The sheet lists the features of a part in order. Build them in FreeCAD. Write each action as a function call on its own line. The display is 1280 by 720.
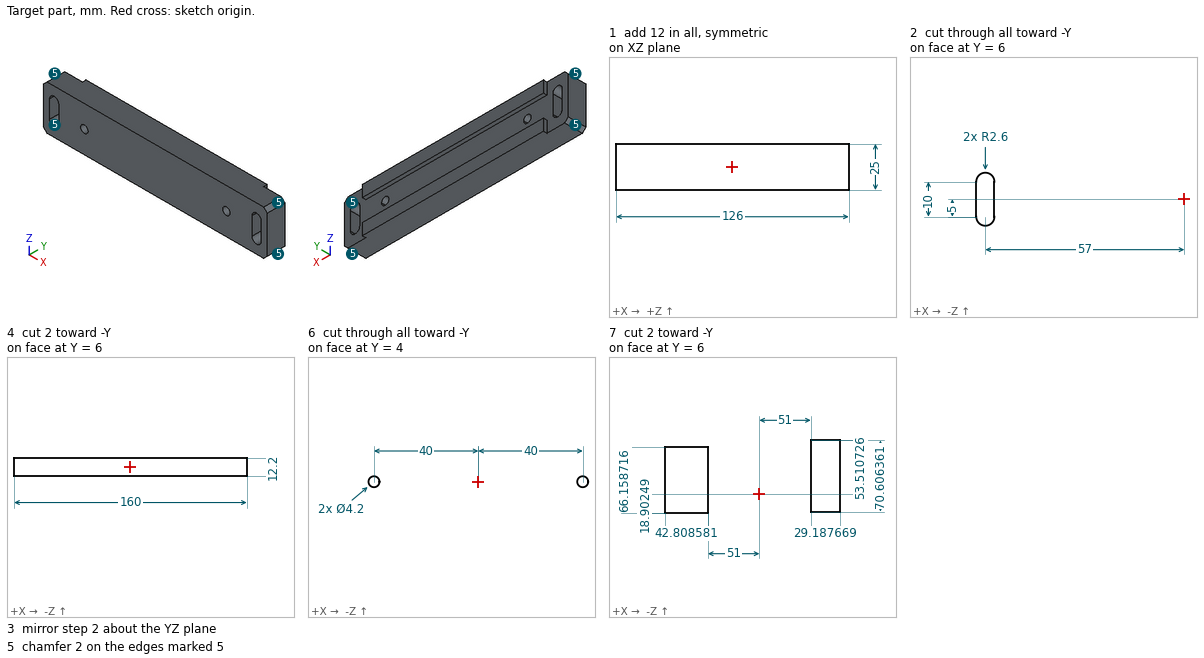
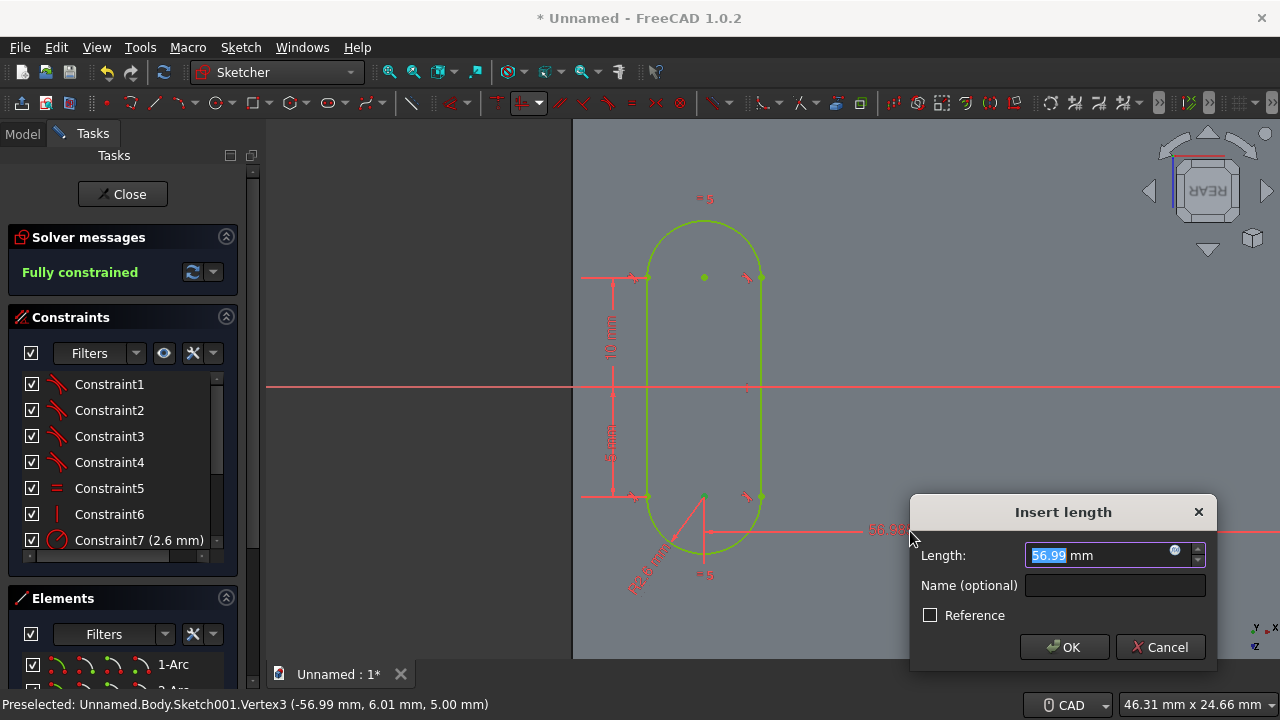
text(57)
key(Return)
key(Escape)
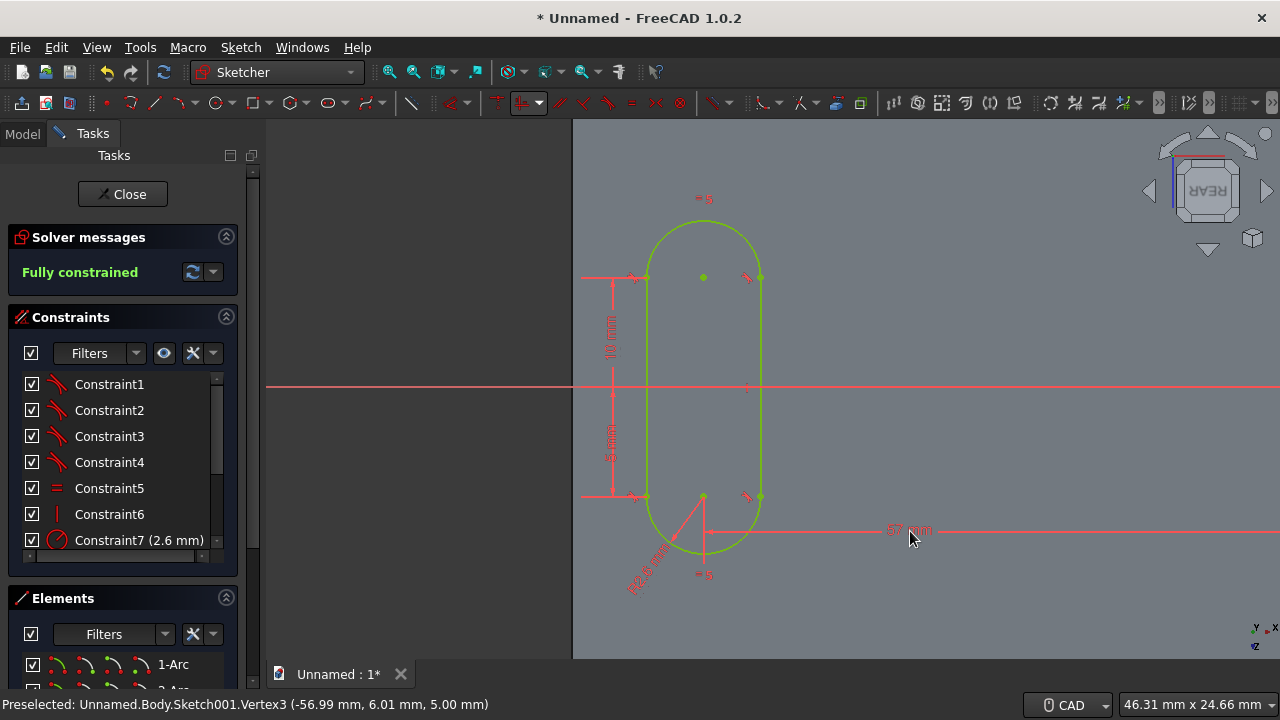
click(123, 194)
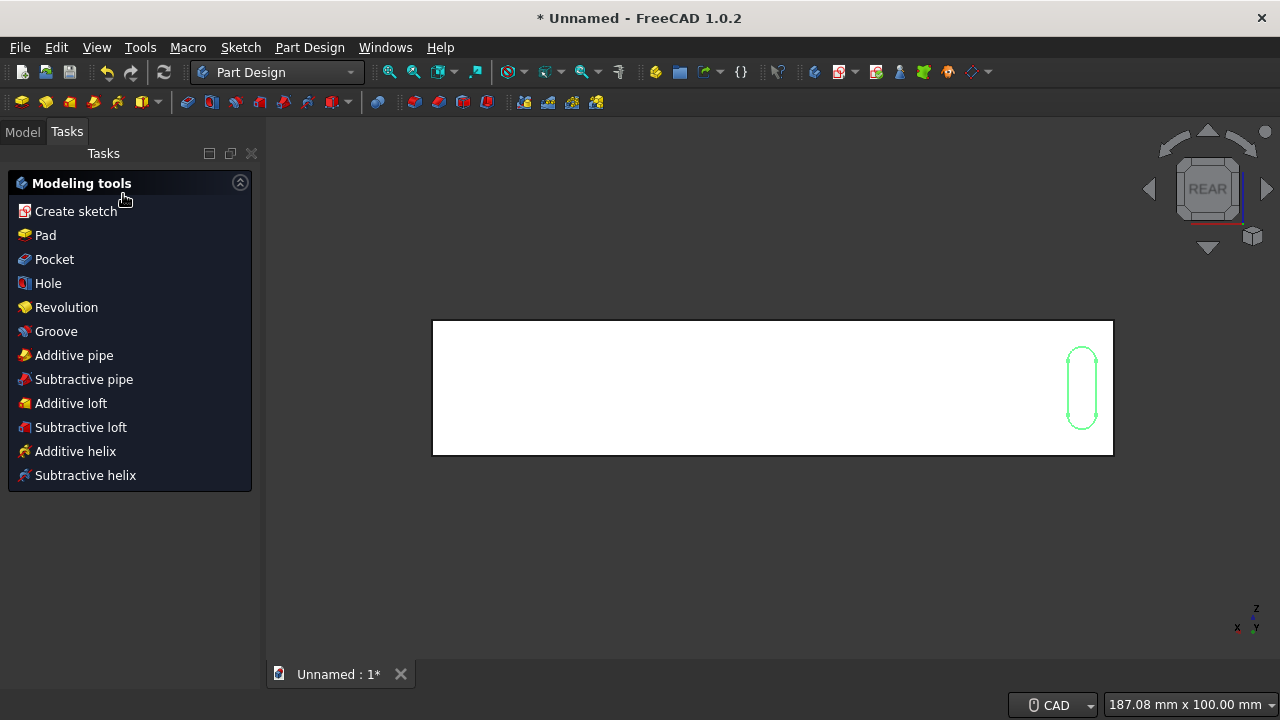
click(188, 102)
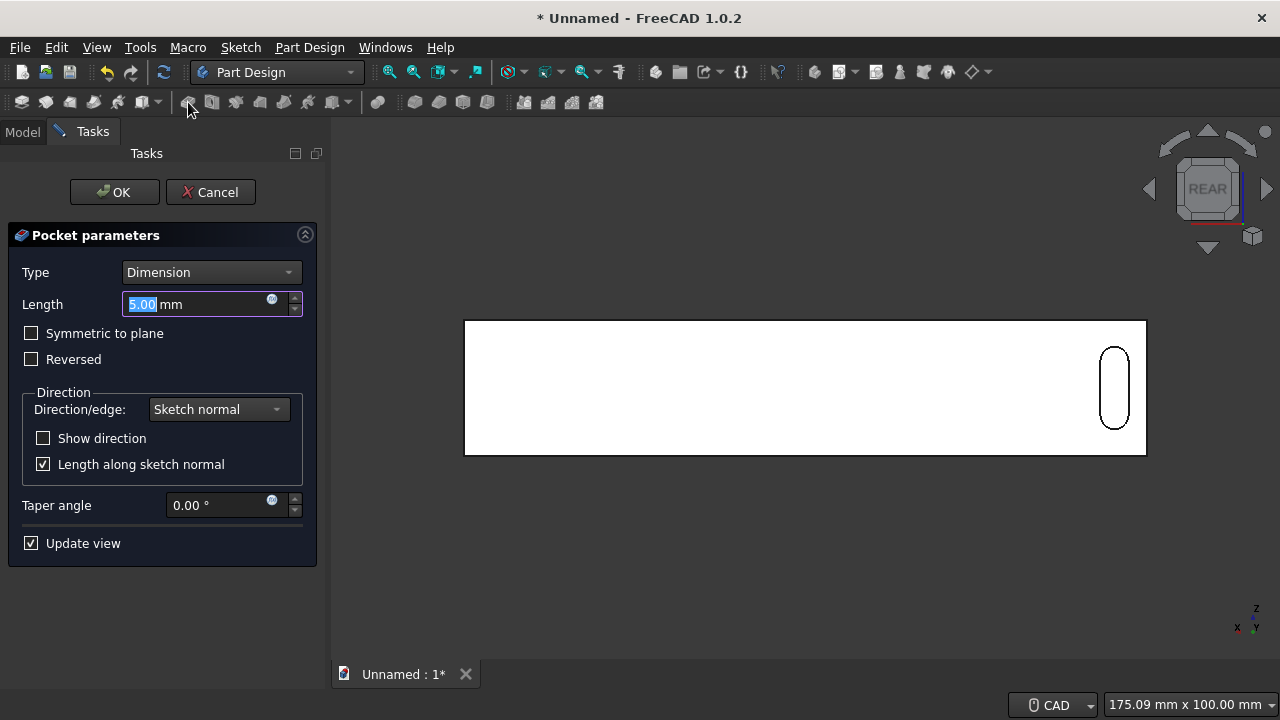
click(212, 272)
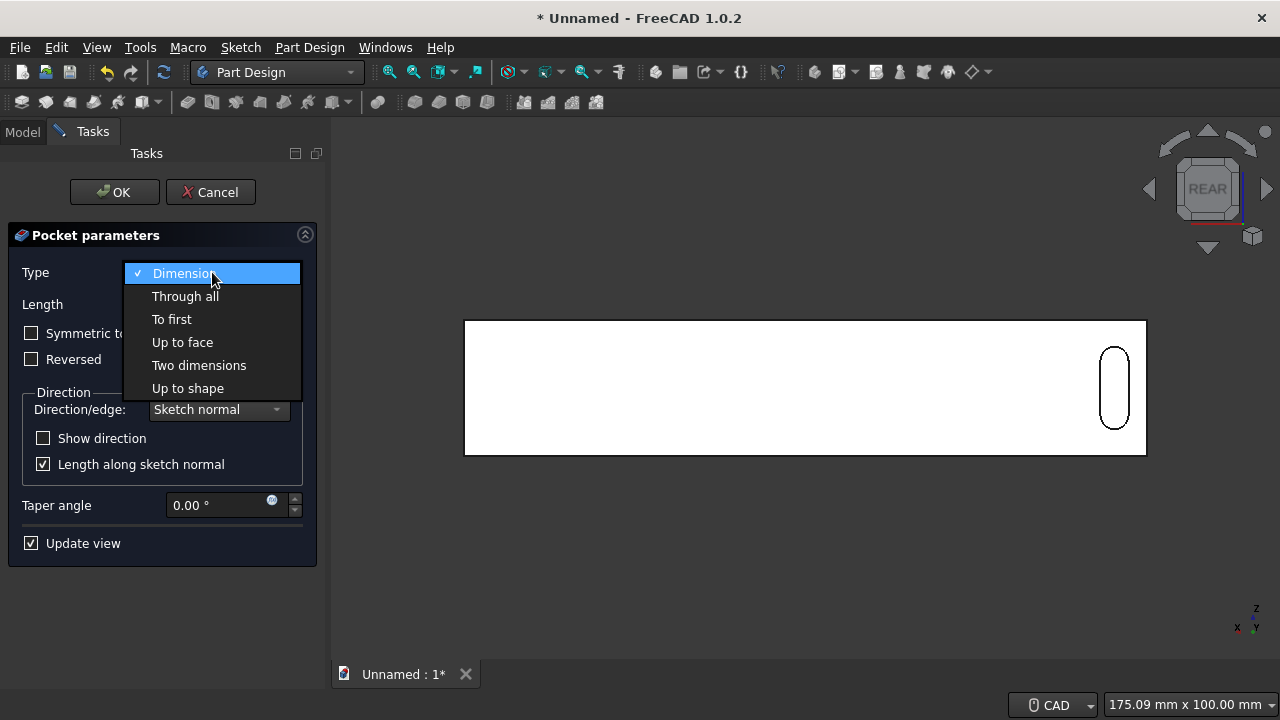
click(212, 296)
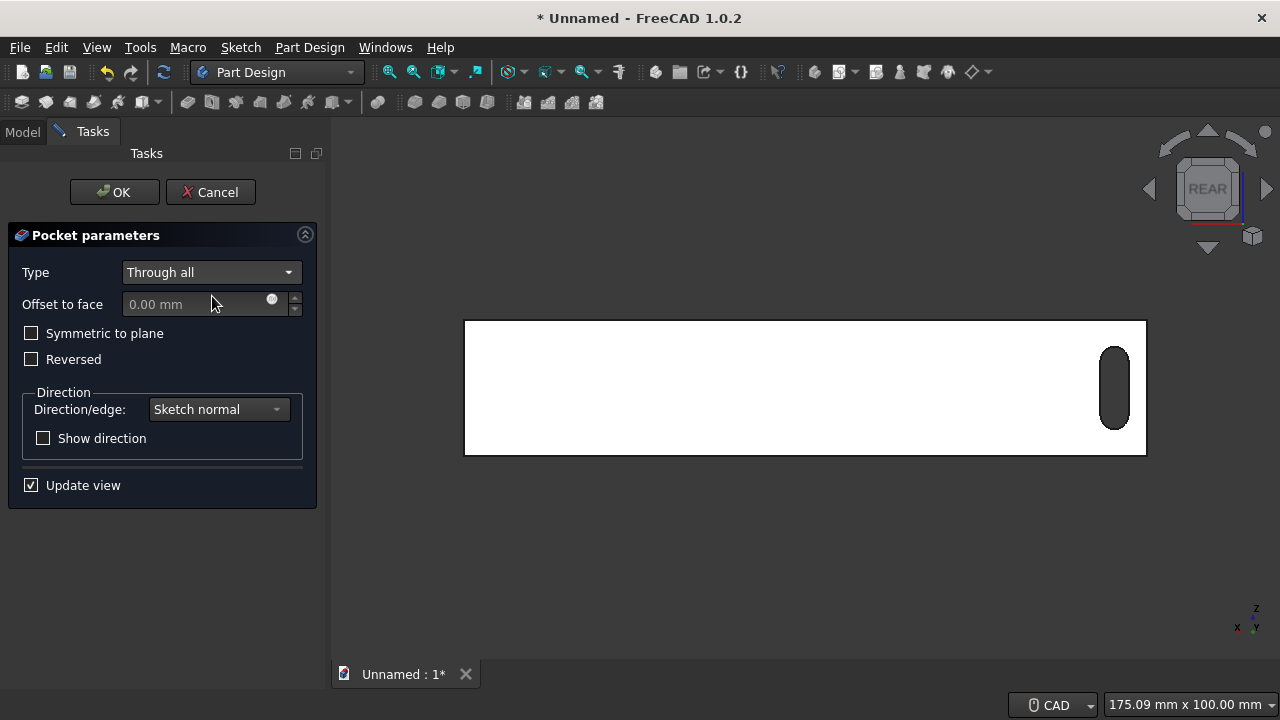
click(115, 192)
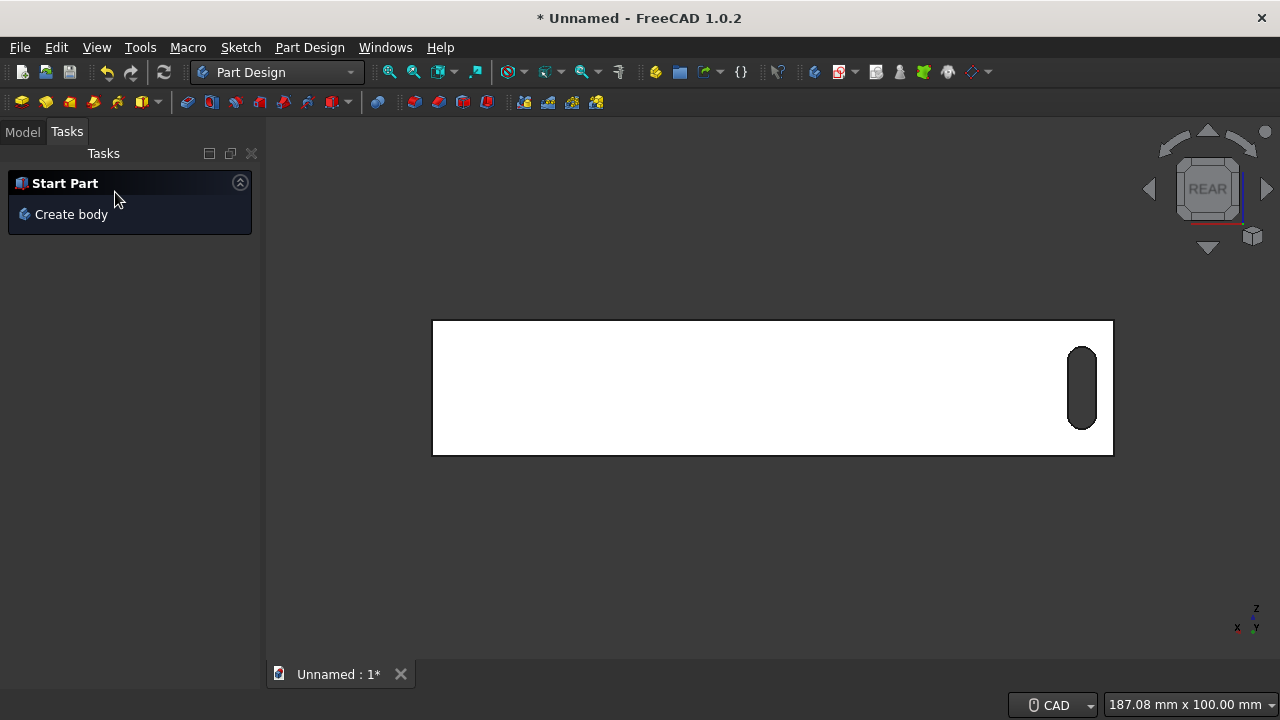
click(23, 131)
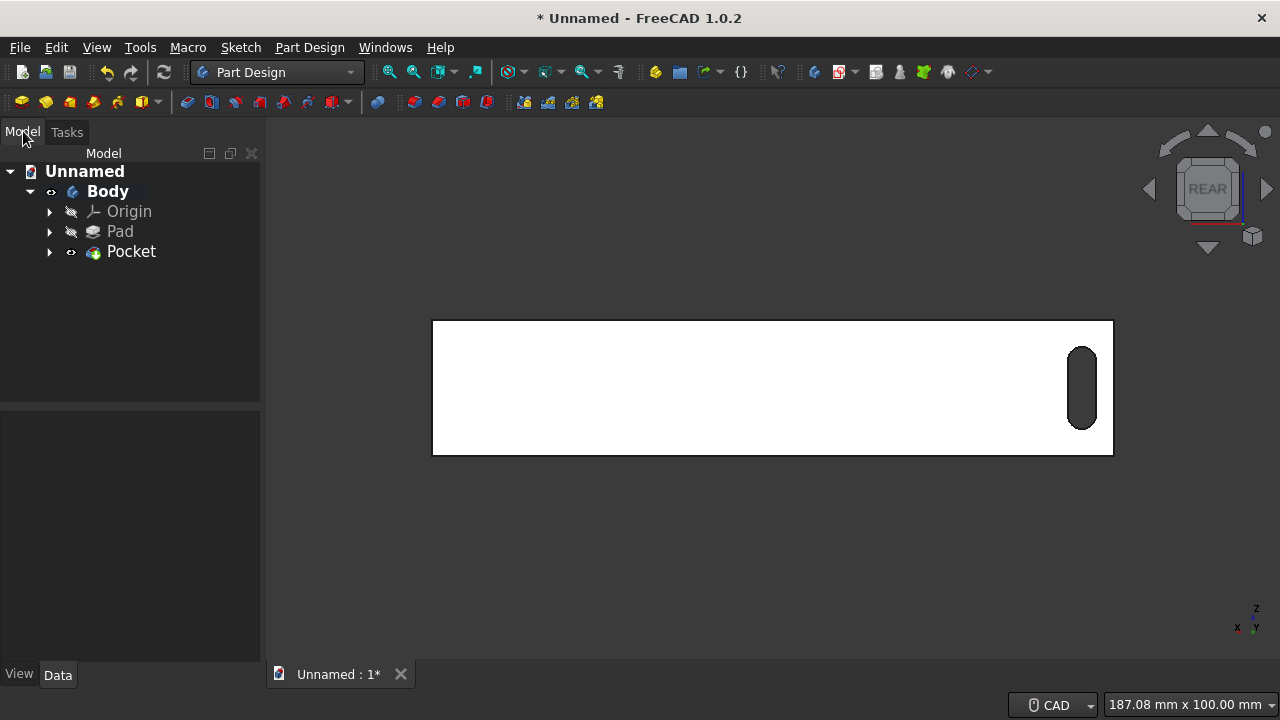
click(116, 252)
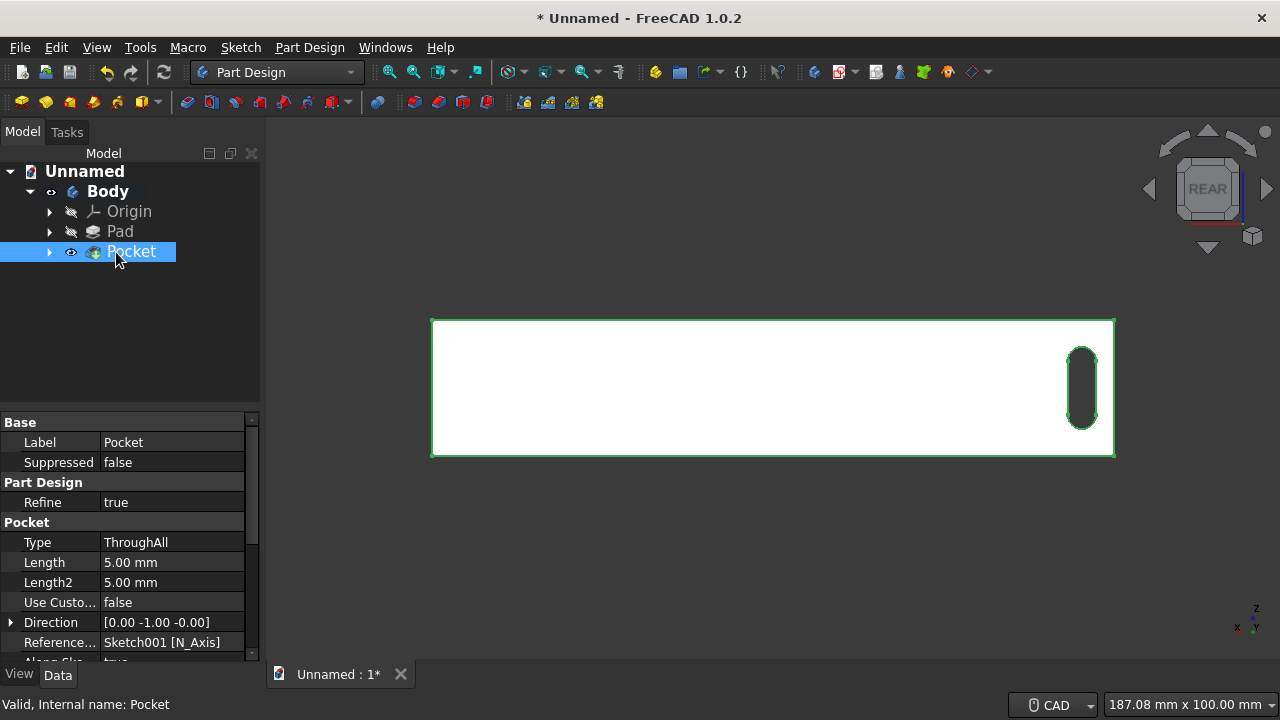
click(524, 102)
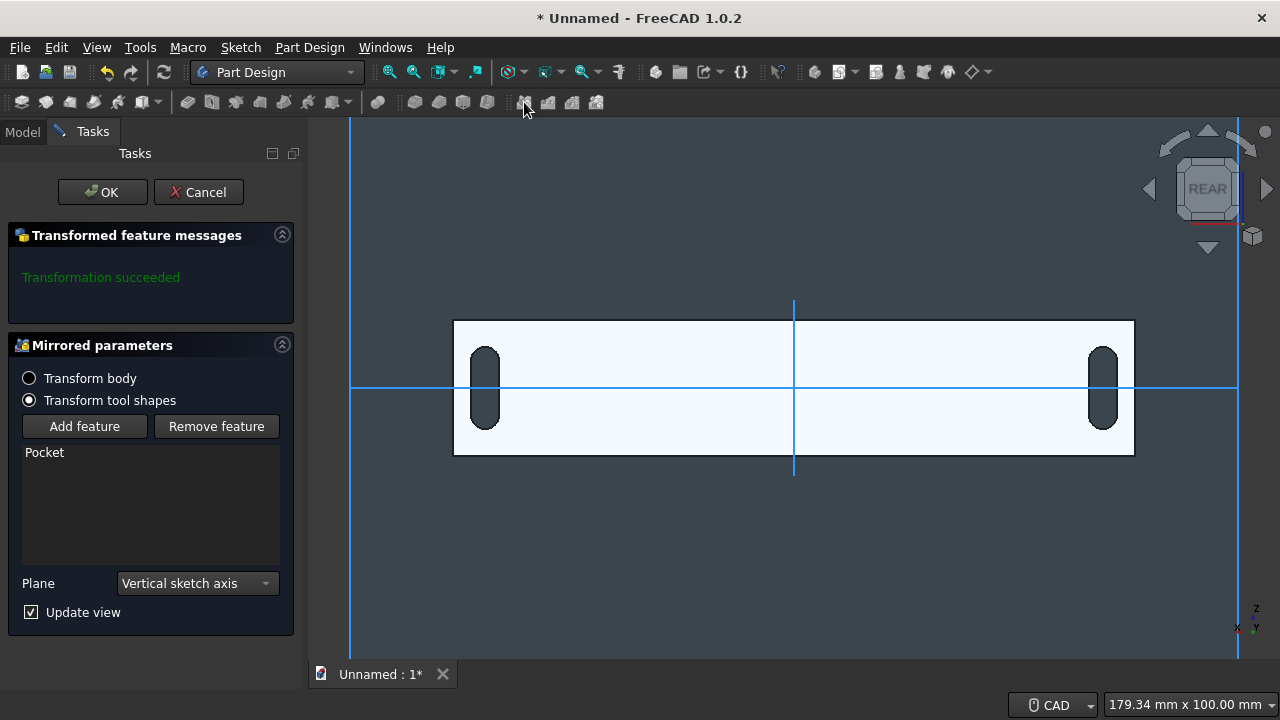
click(198, 584)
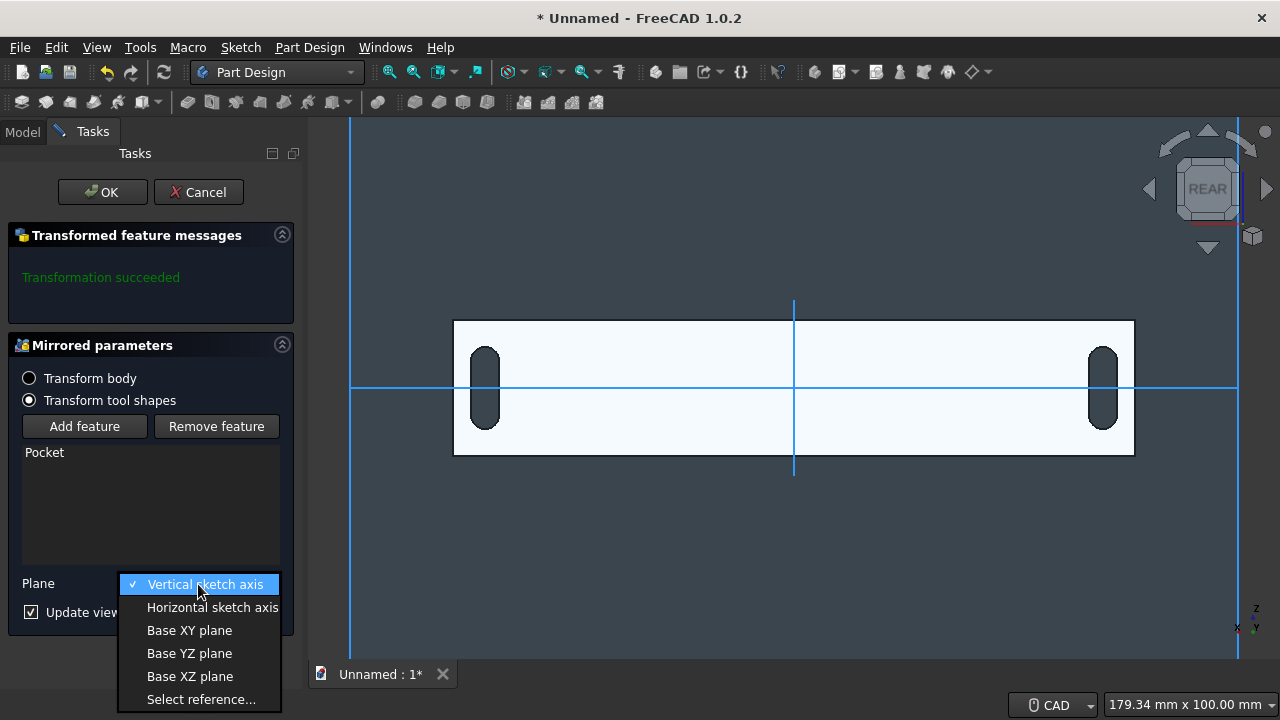
click(198, 654)